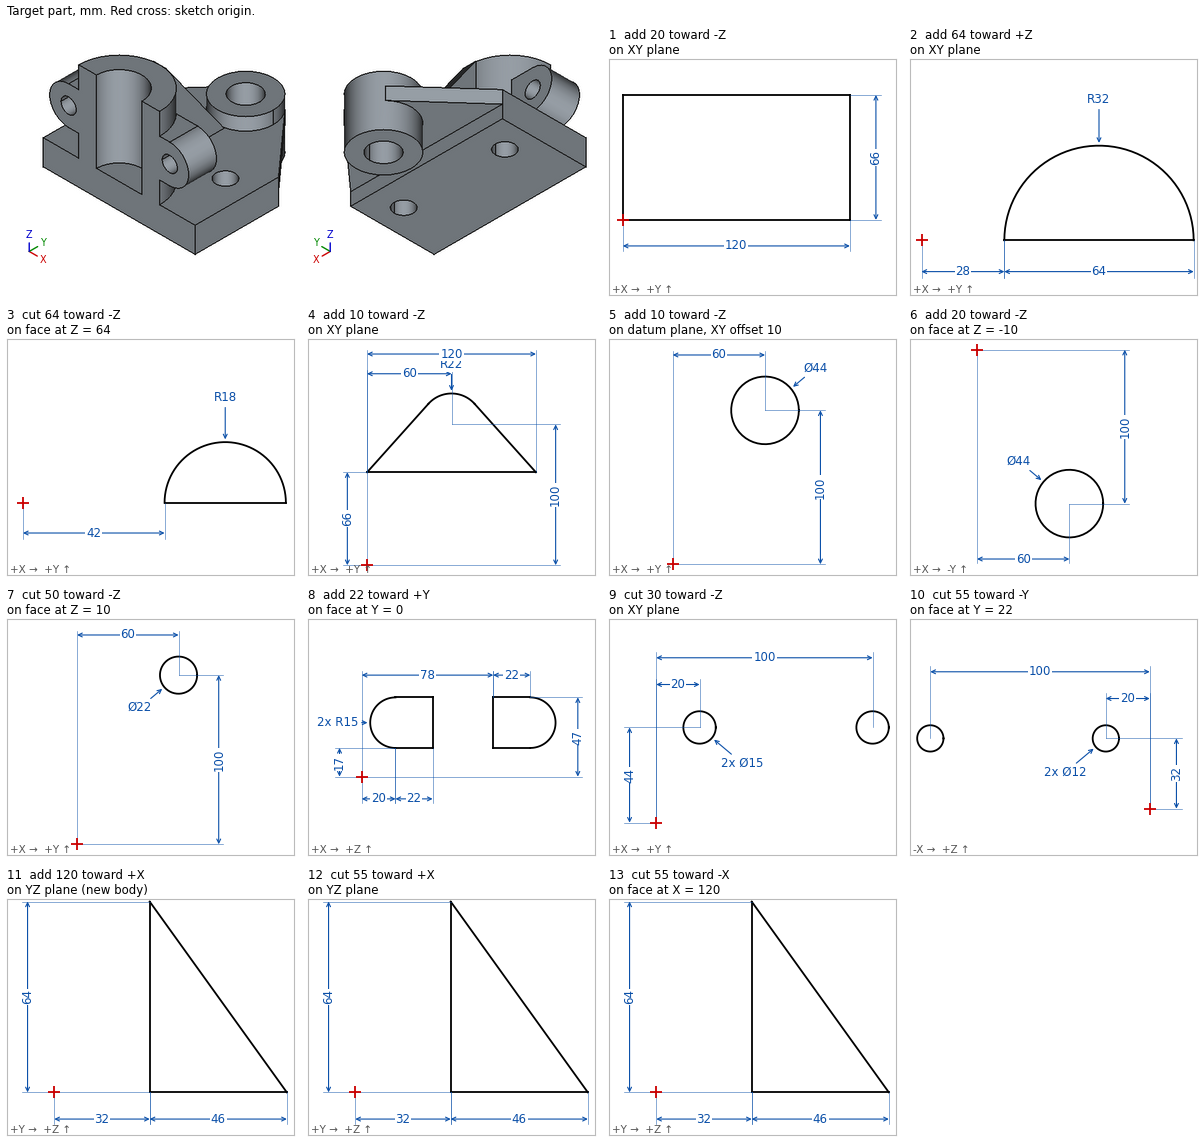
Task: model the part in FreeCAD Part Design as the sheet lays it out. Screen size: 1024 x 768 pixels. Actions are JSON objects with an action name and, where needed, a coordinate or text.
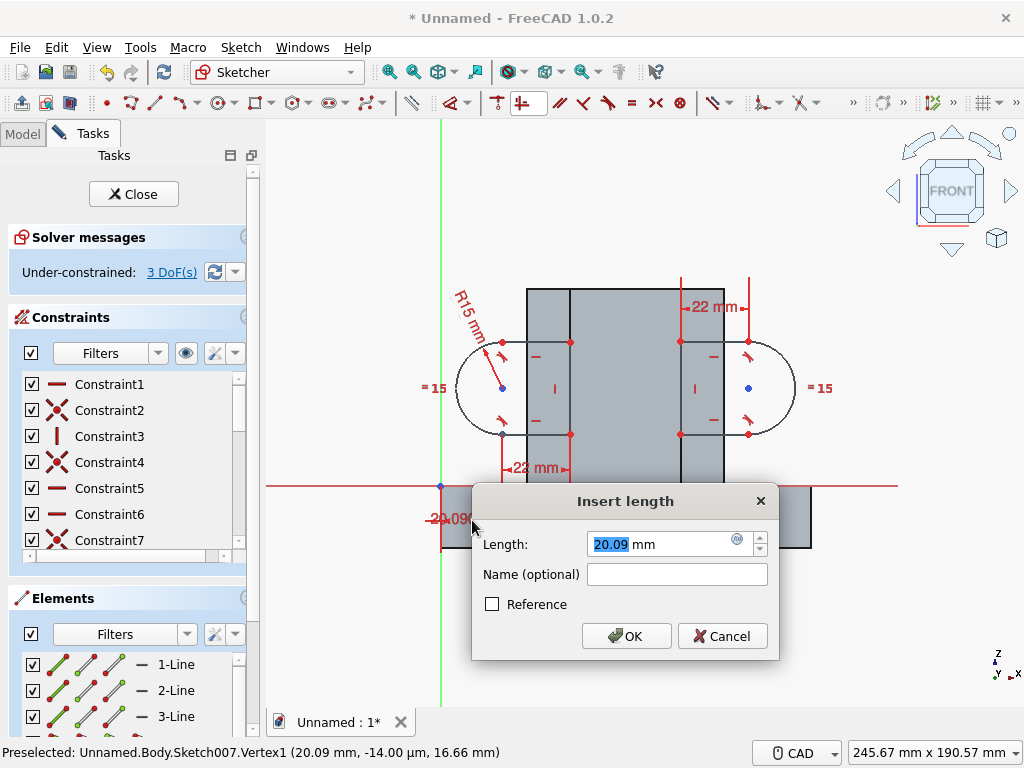
{"action": "type", "text": "20"}
{"action": "key", "text": "Return"}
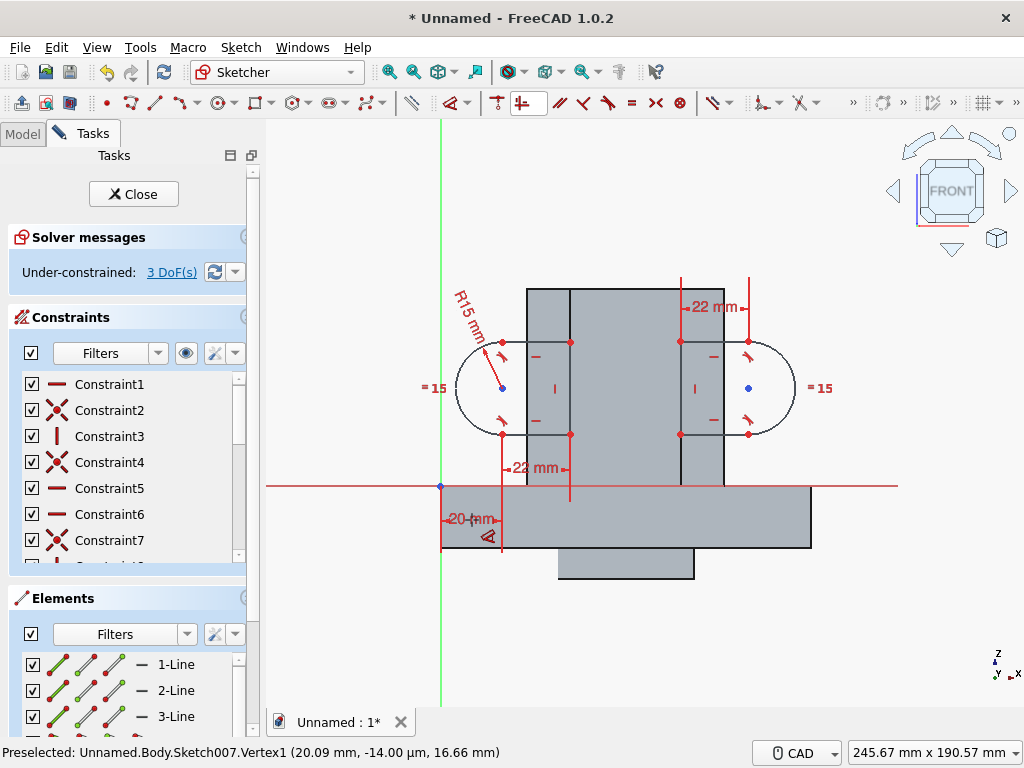
{"action": "left_click", "coordinate": [502, 435]}
{"action": "left_click", "coordinate": [407, 460]}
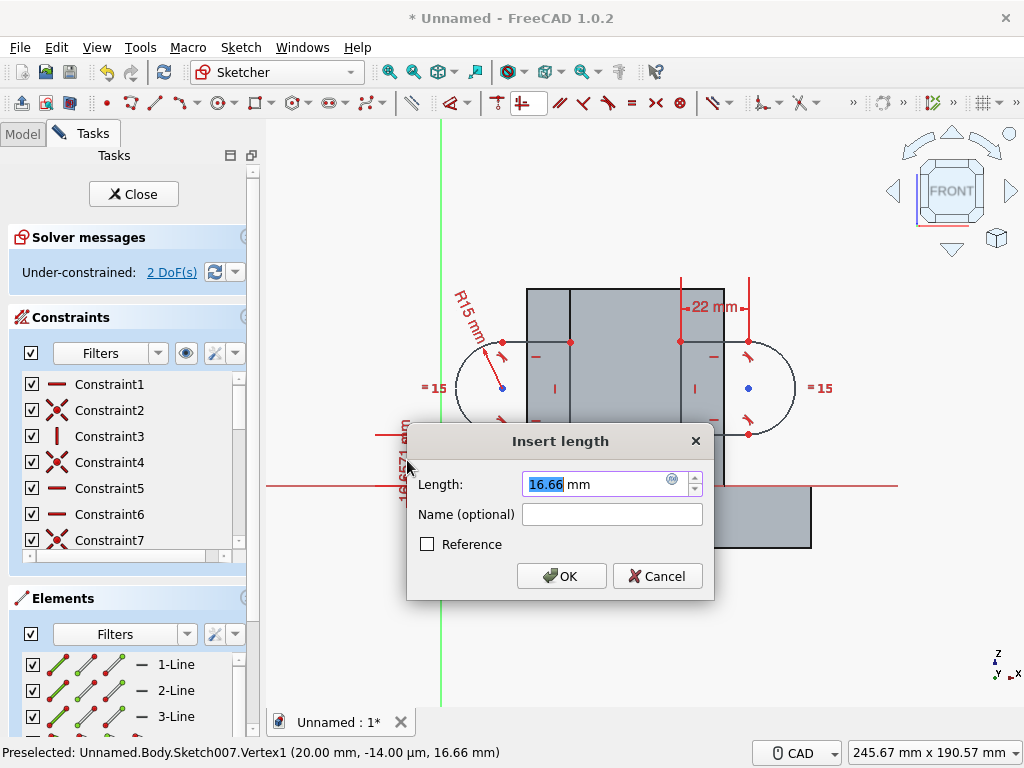
{"action": "type", "text": "17"}
{"action": "key", "text": "Return"}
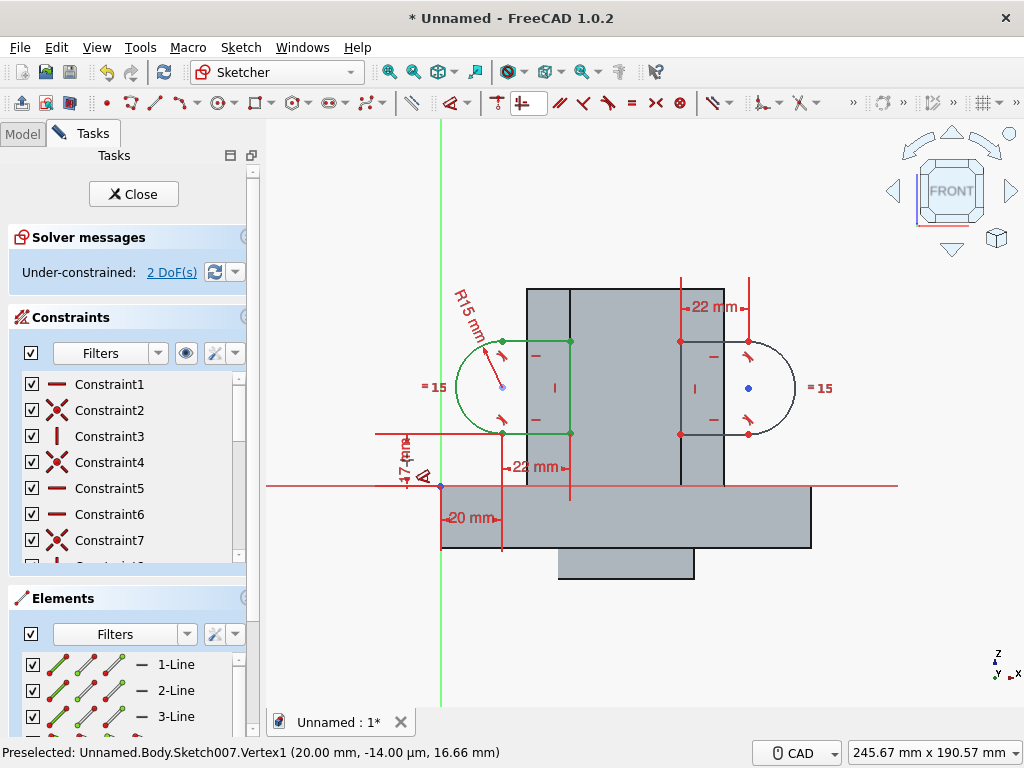
{"action": "left_click", "coordinate": [749, 342]}
{"action": "left_click", "coordinate": [407, 414]}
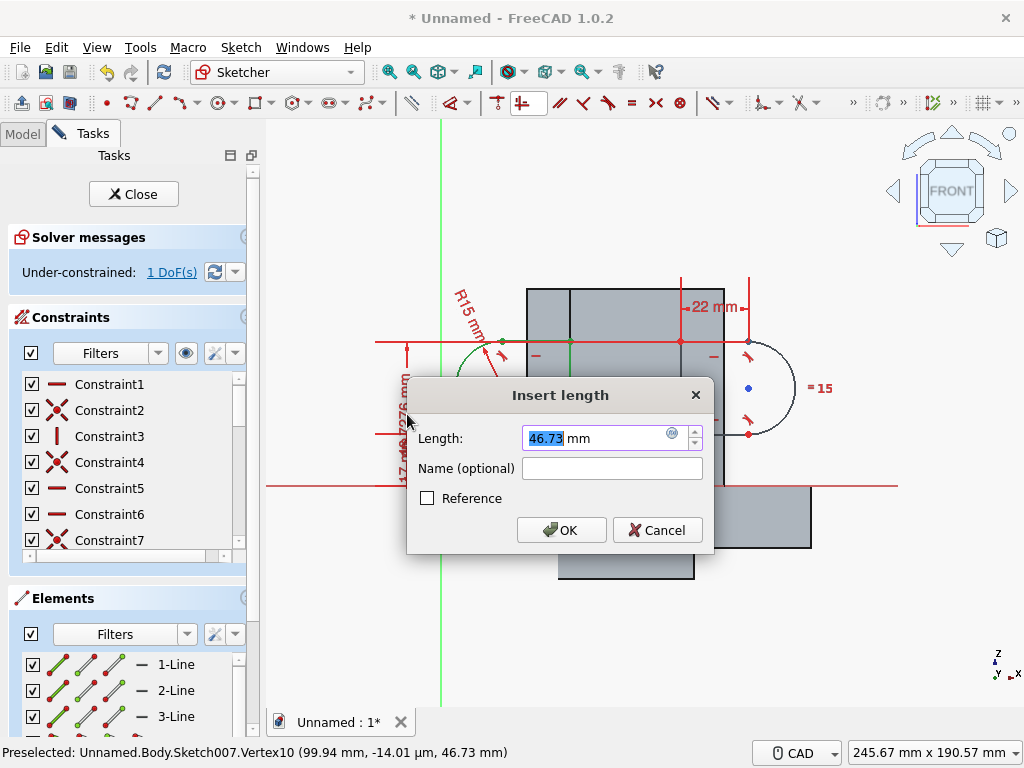
{"action": "type", "text": "47"}
{"action": "key", "text": "Return"}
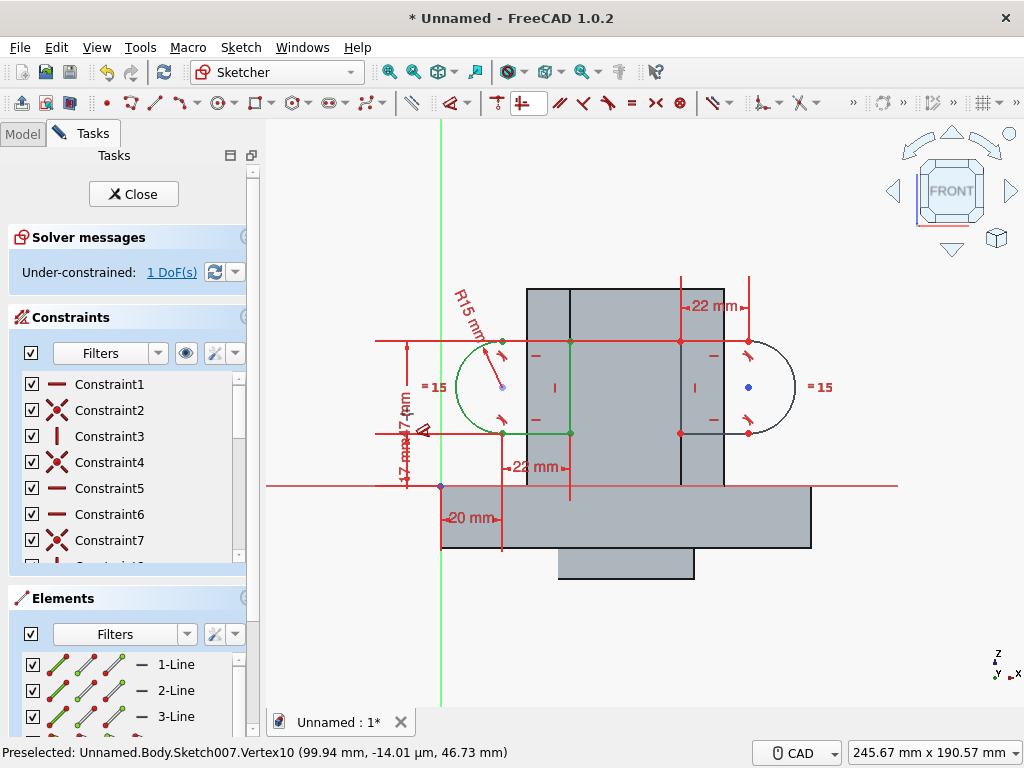
{"action": "left_click", "coordinate": [681, 341]}
{"action": "left_click", "coordinate": [561, 520]}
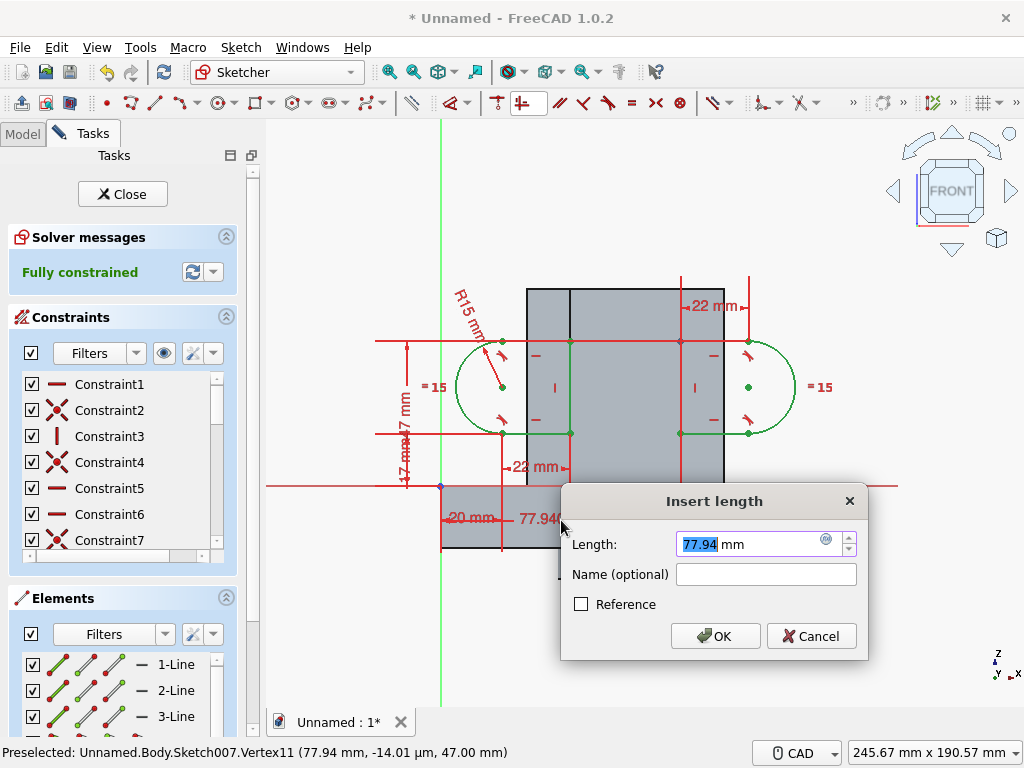
{"action": "type", "text": "78"}
{"action": "key", "text": "Return"}
{"action": "key", "text": "Escape"}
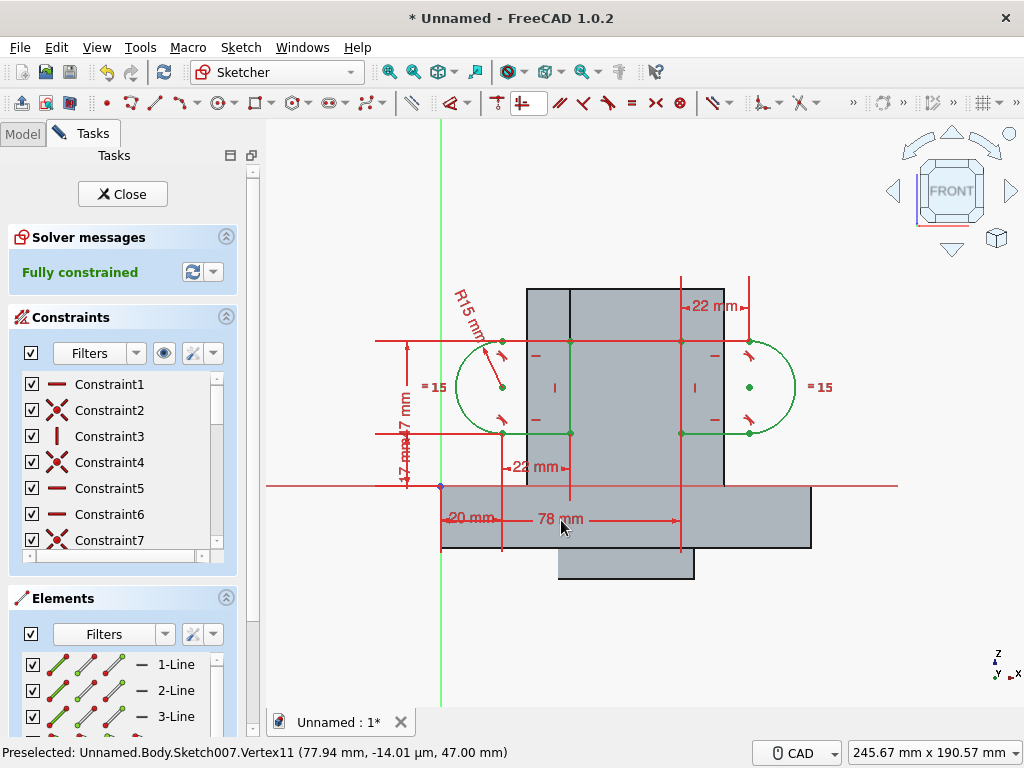
{"action": "left_click", "coordinate": [123, 194]}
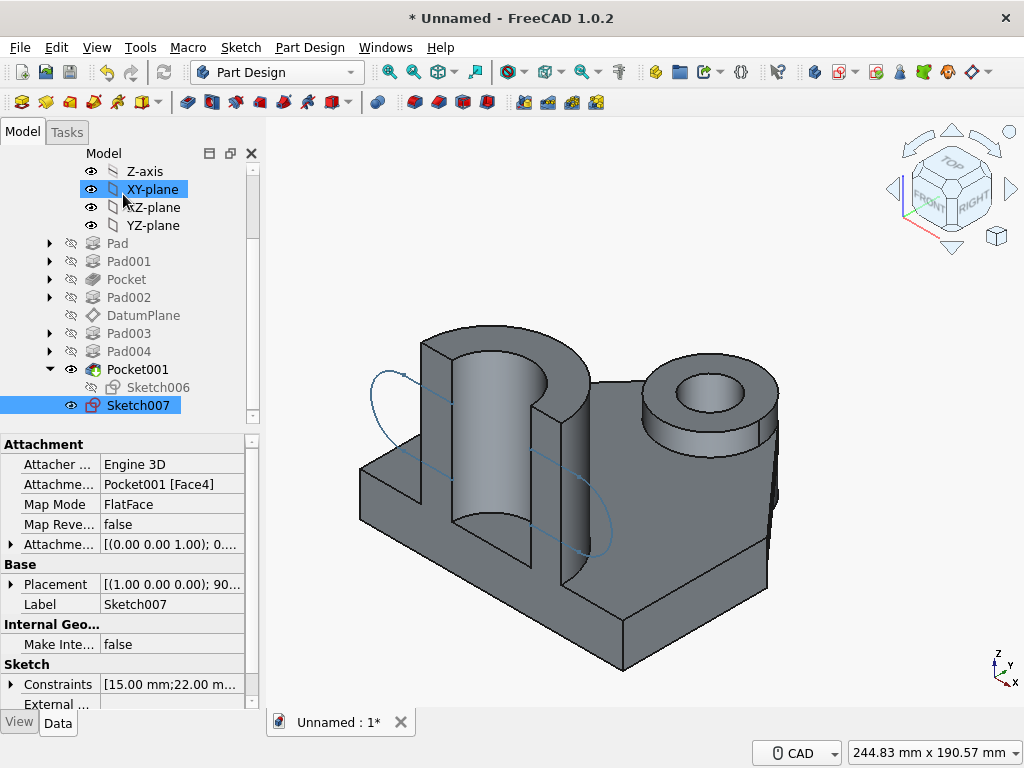
{"action": "left_click", "coordinate": [22, 102]}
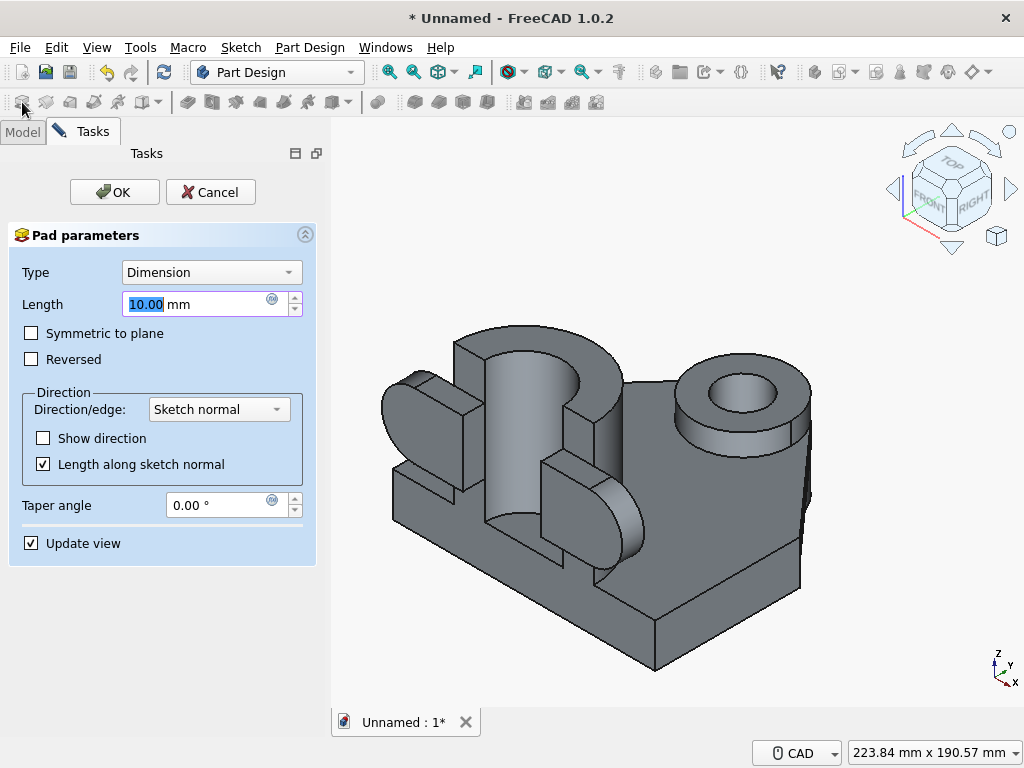
{"action": "type", "text": "22"}
{"action": "key", "text": "Tab"}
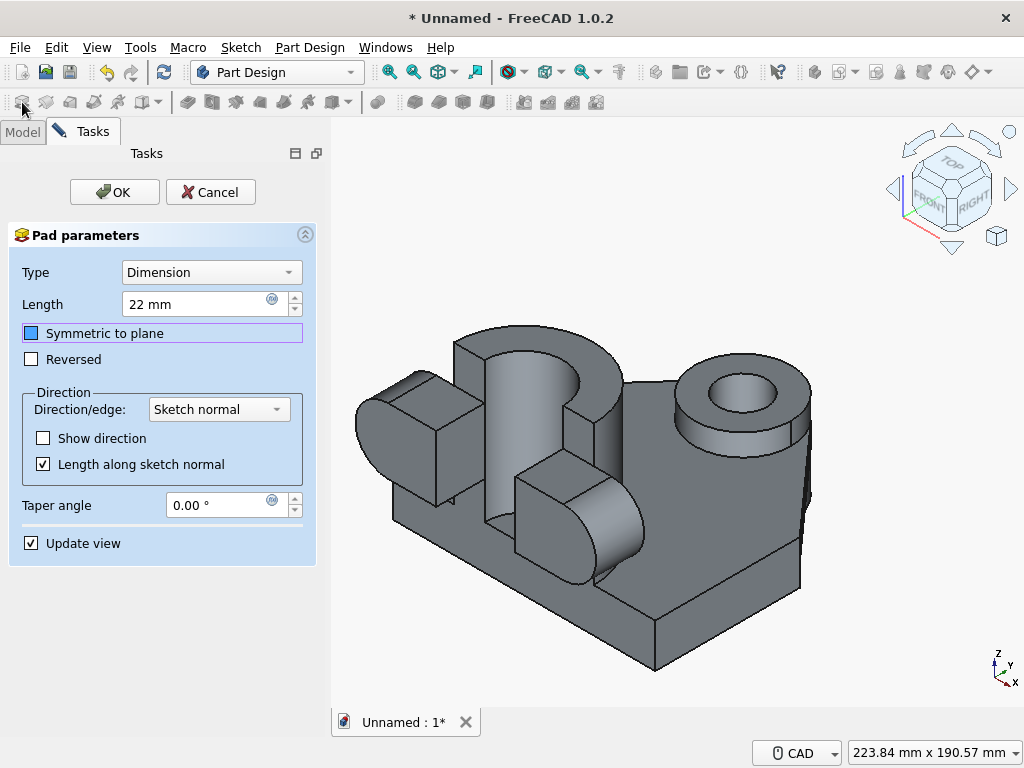
{"action": "left_click", "coordinate": [30, 359]}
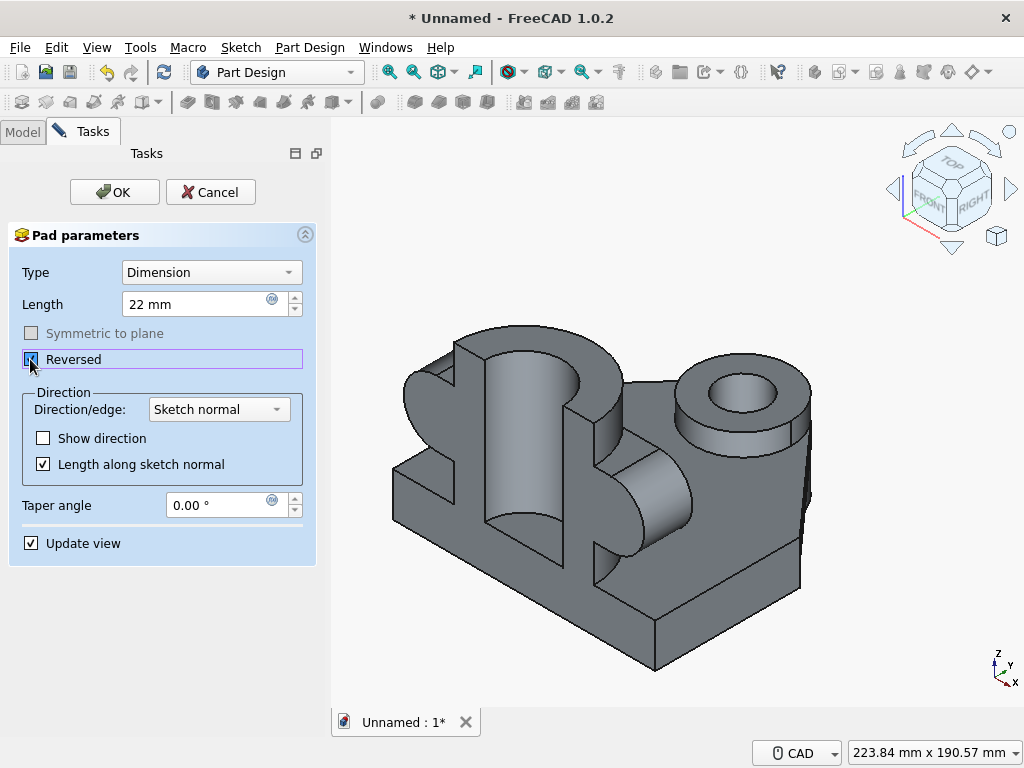
{"action": "left_click", "coordinate": [115, 192]}